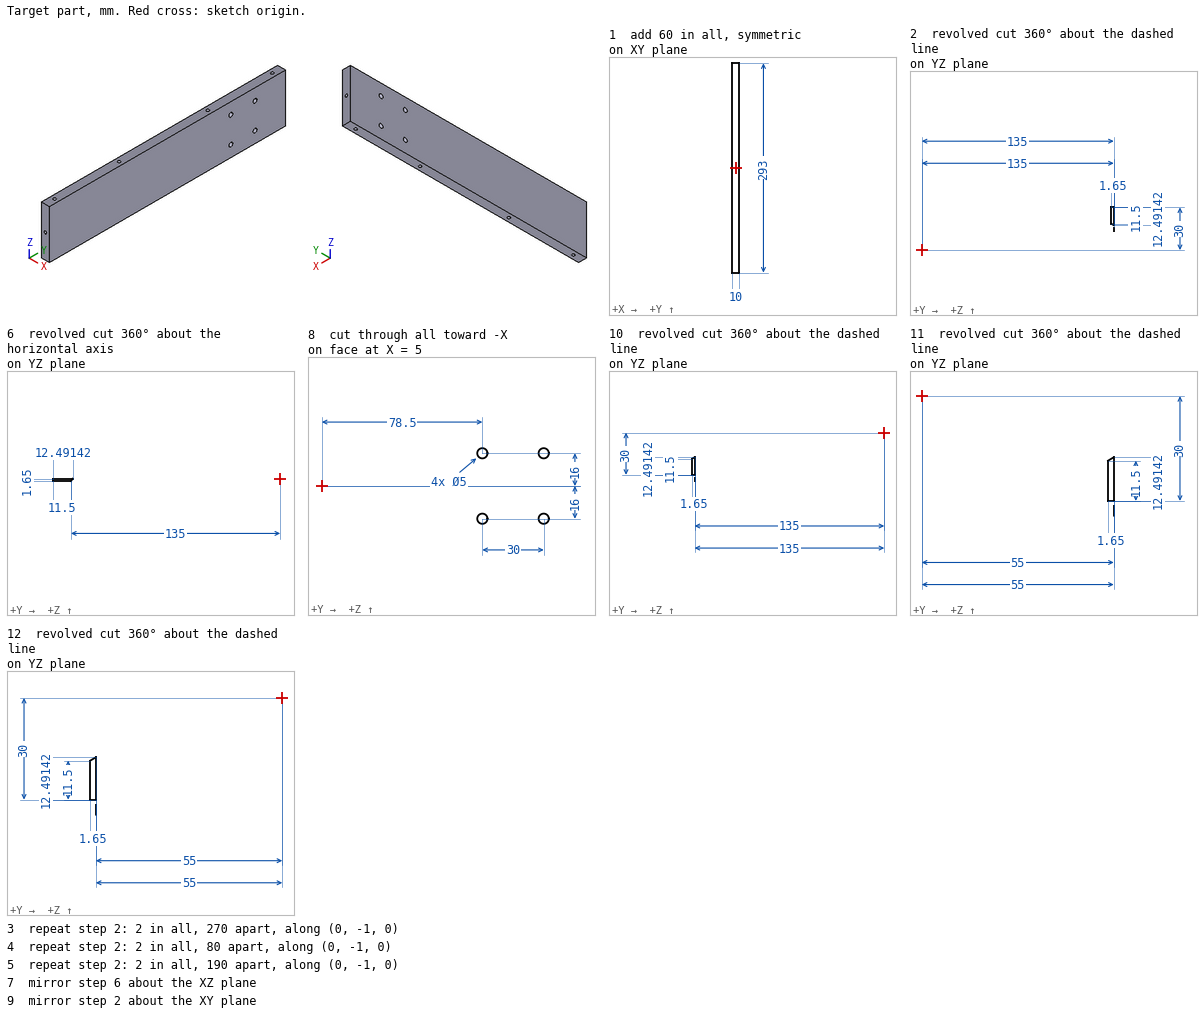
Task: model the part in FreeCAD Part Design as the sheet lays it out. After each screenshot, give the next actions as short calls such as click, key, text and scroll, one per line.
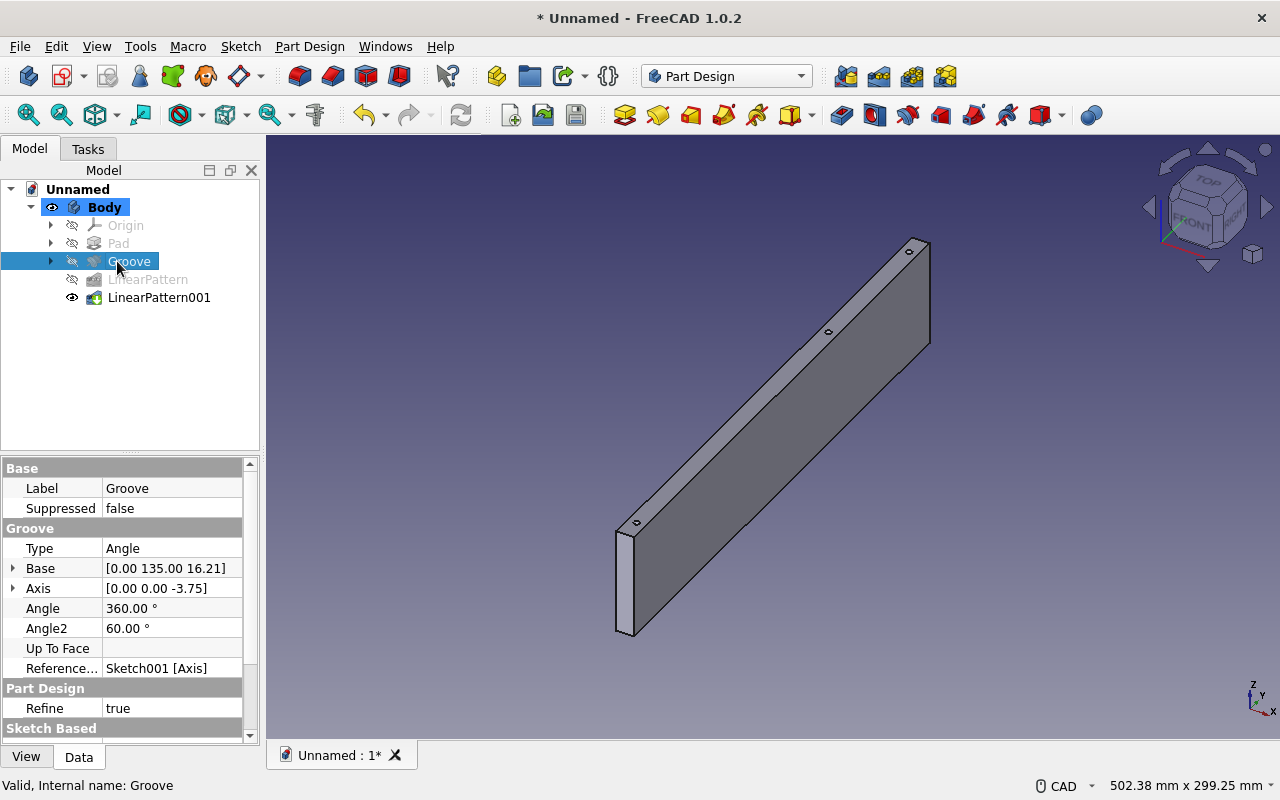
click(879, 76)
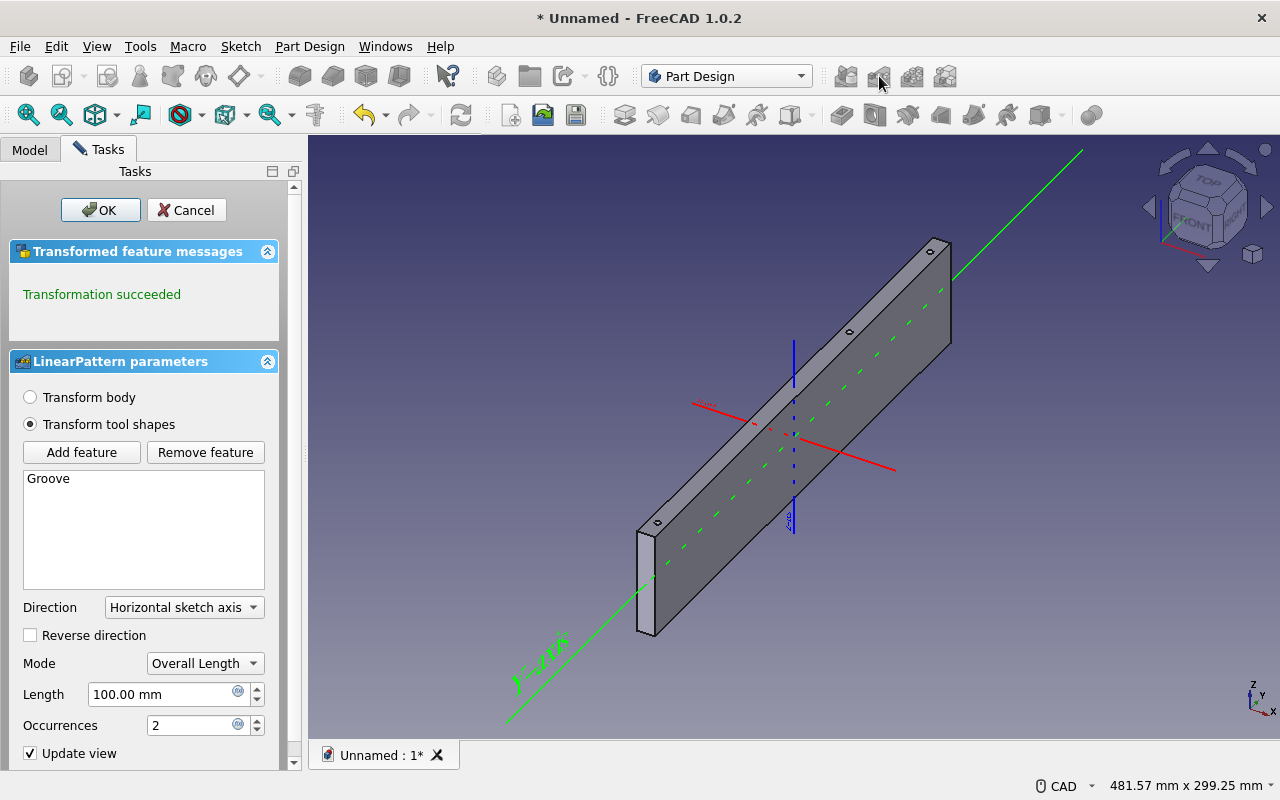
click(185, 608)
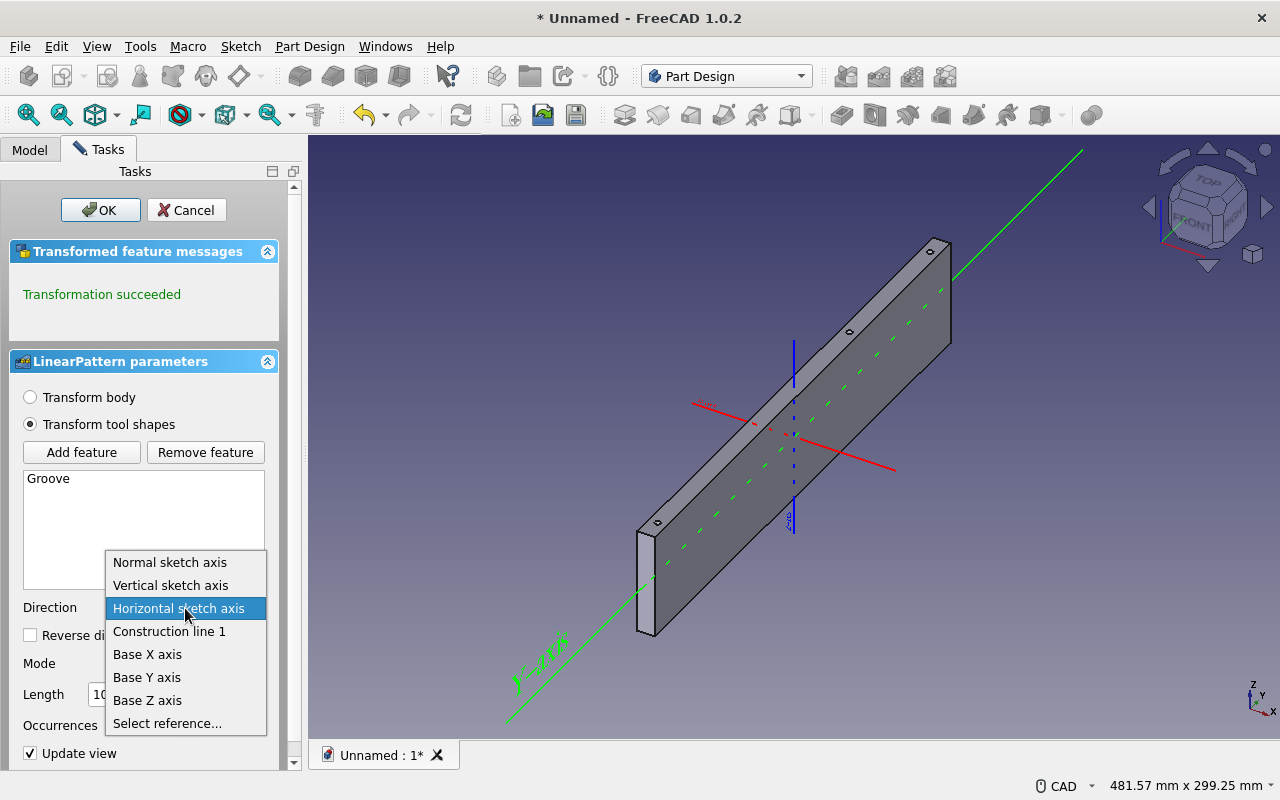
click(184, 678)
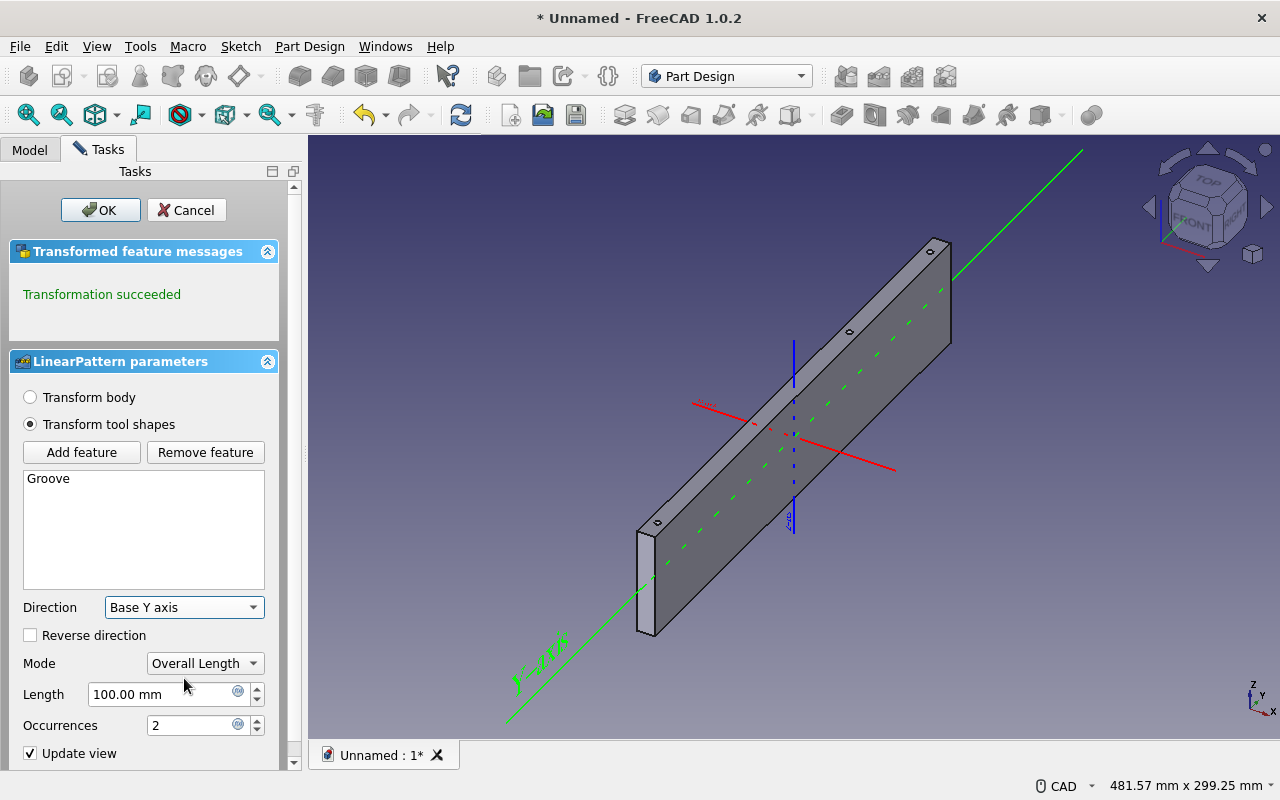
click(206, 664)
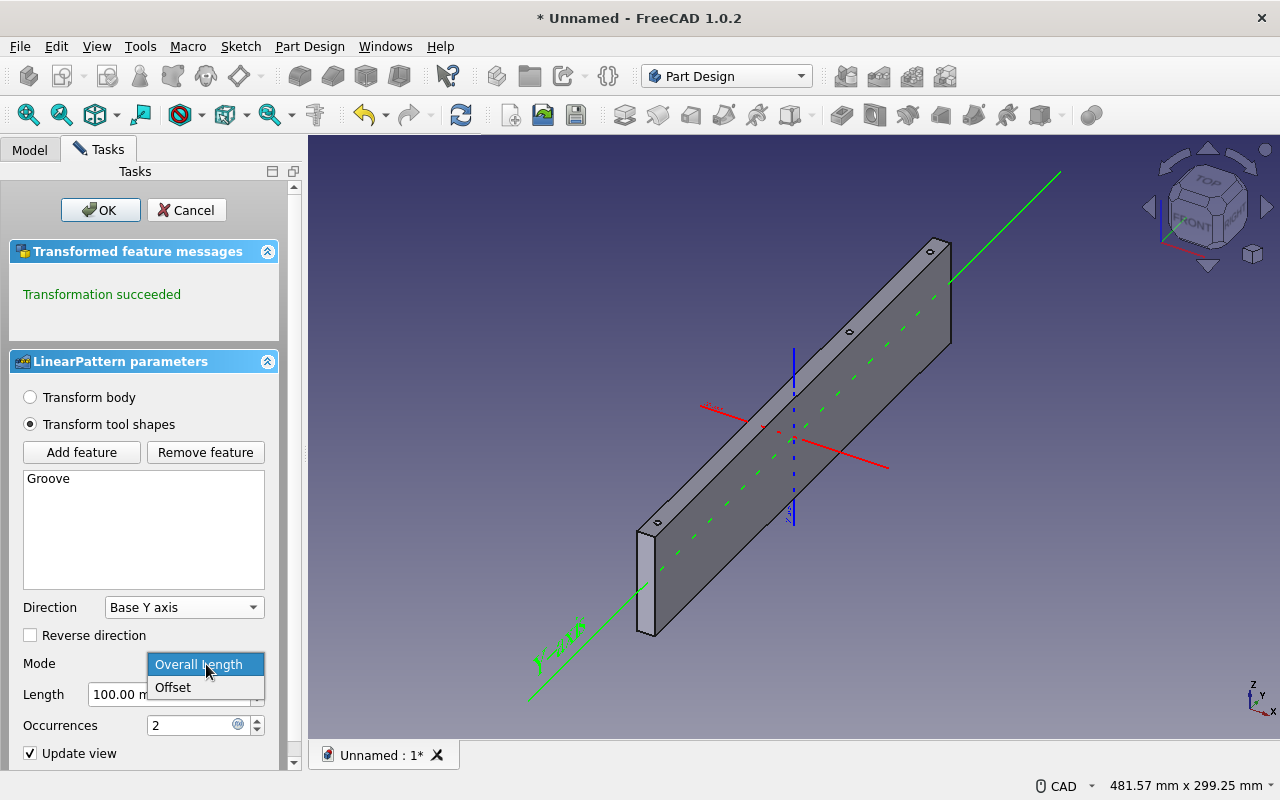
click(204, 688)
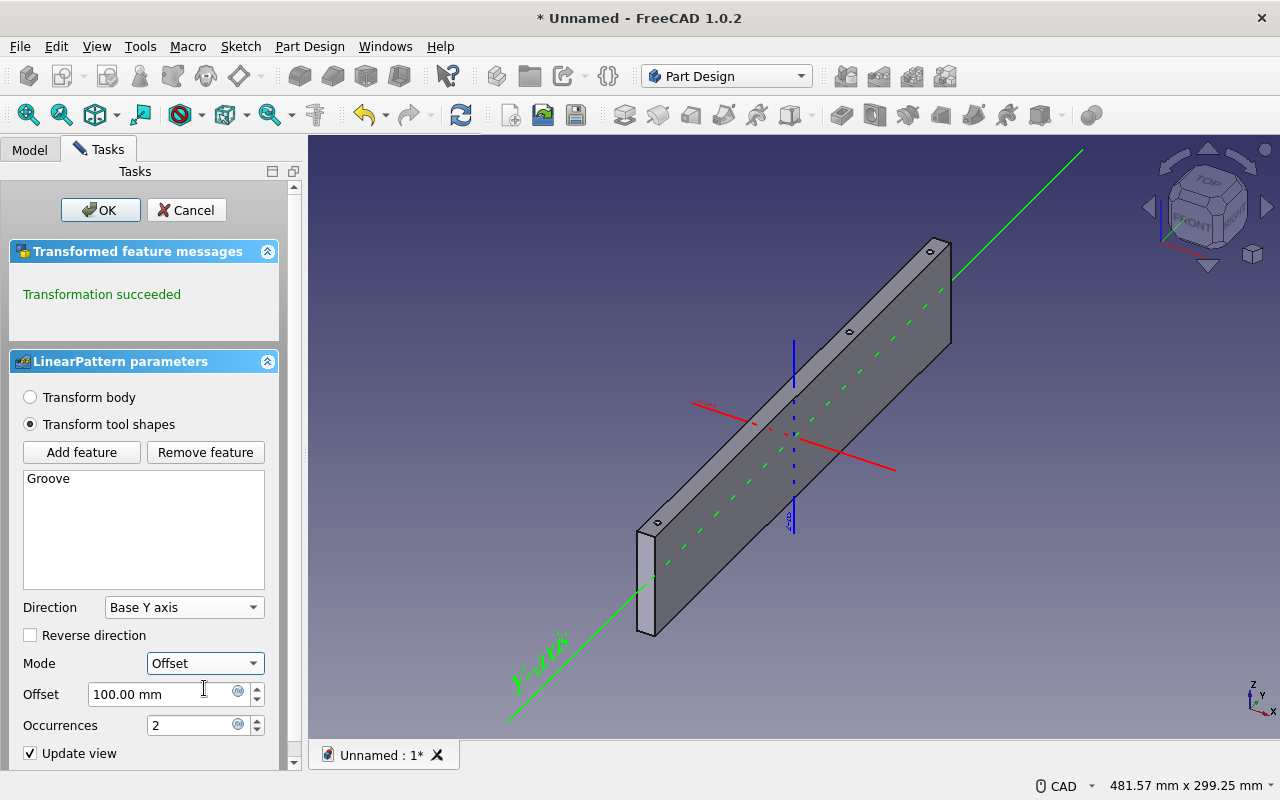
triple_click(170, 694)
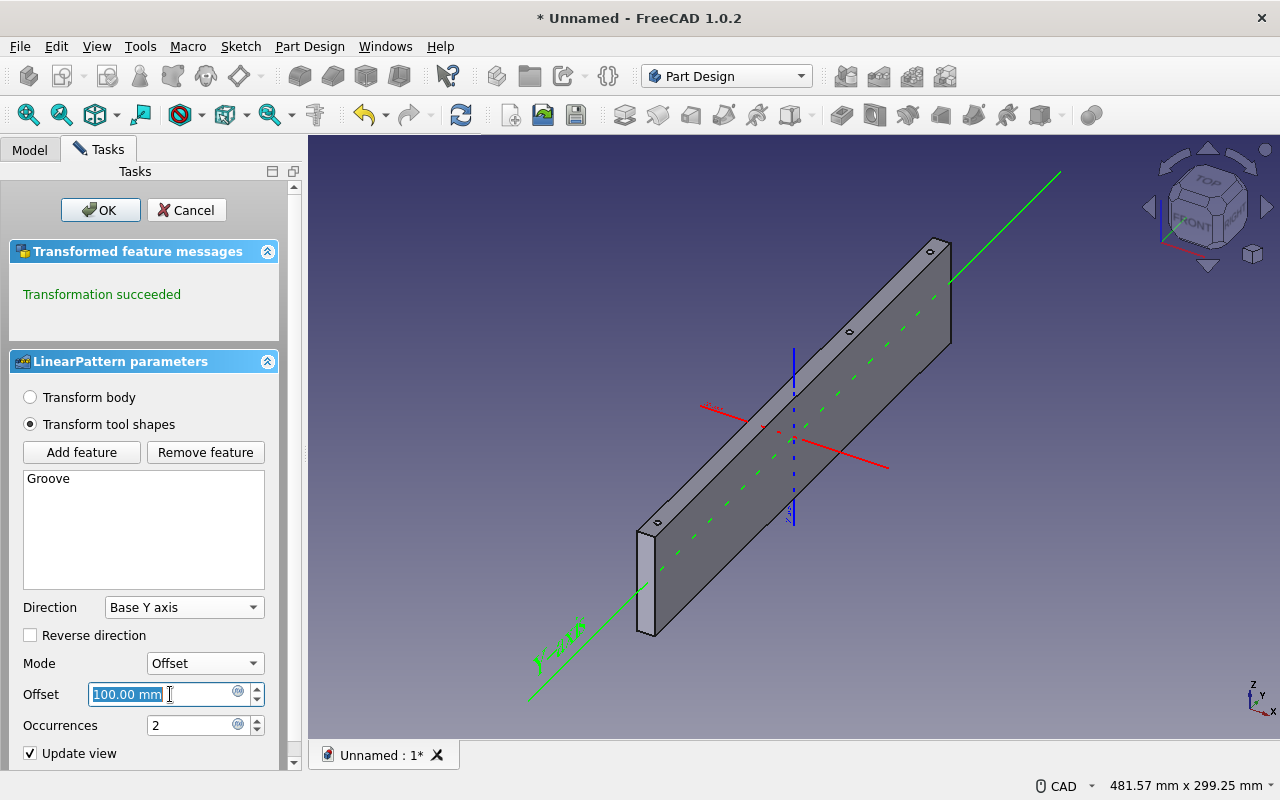
text(190)
key(Tab)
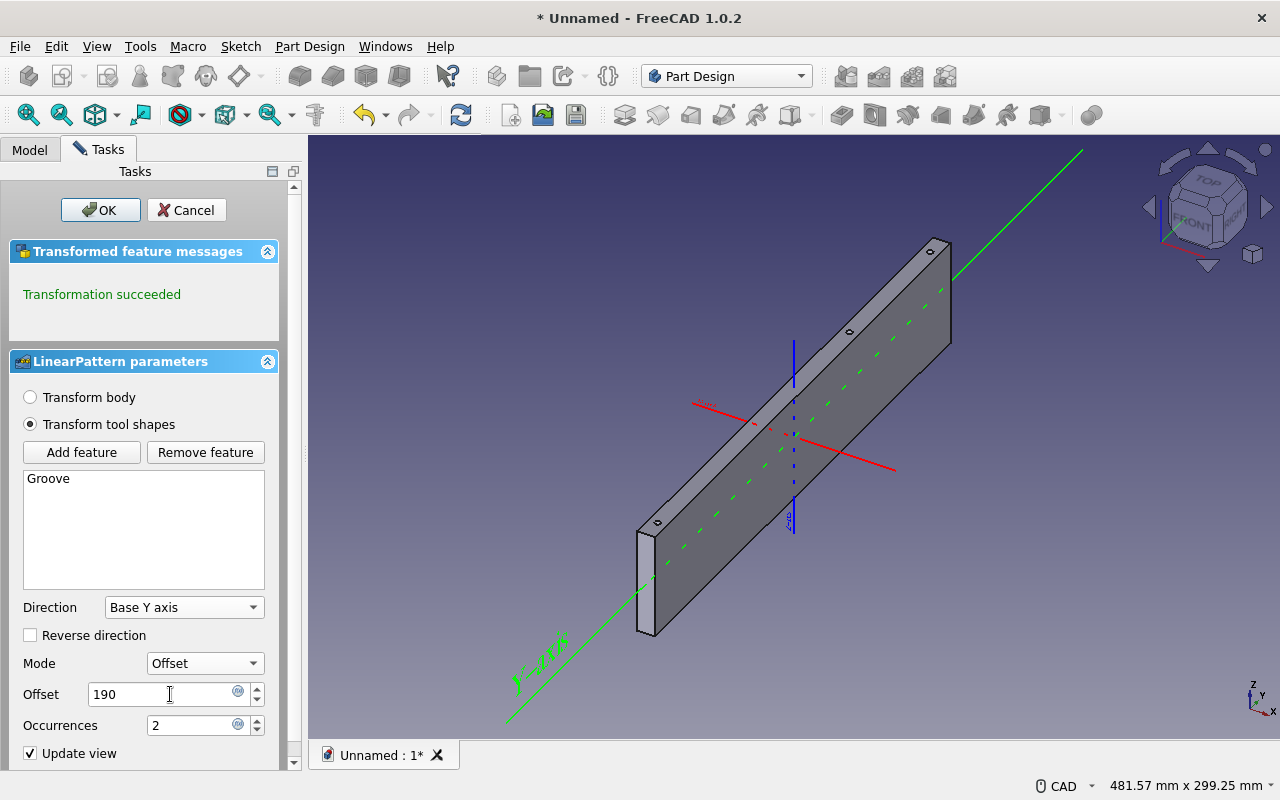
triple_click(199, 726)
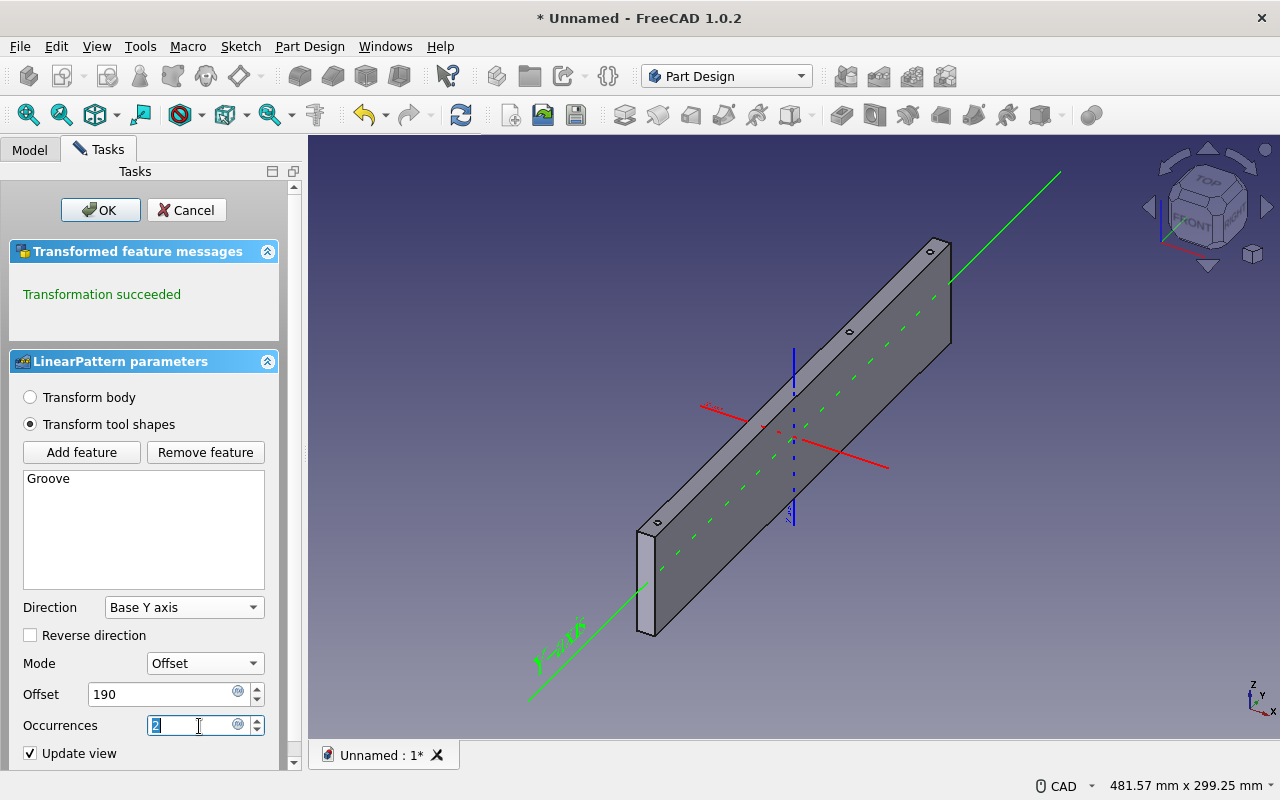
text(2)
key(Tab)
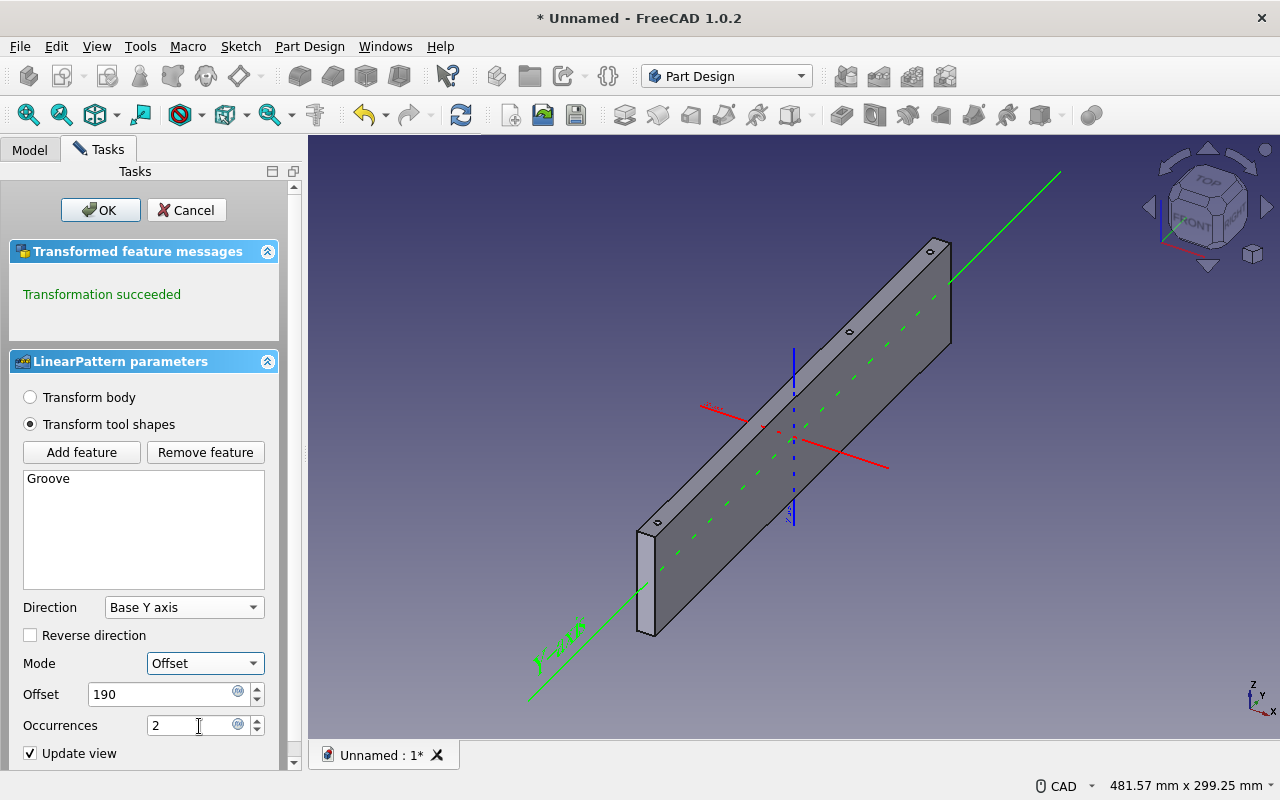
click(31, 635)